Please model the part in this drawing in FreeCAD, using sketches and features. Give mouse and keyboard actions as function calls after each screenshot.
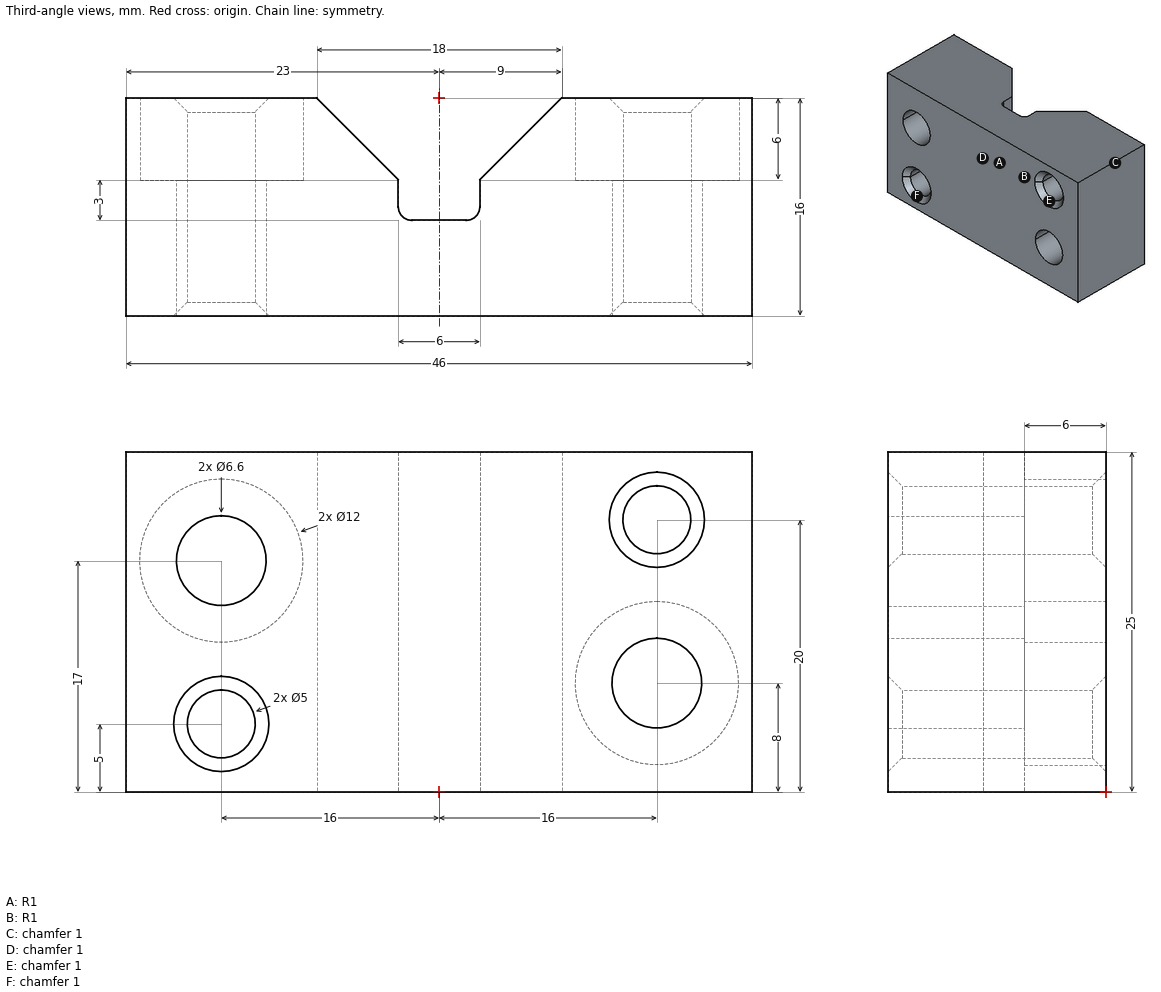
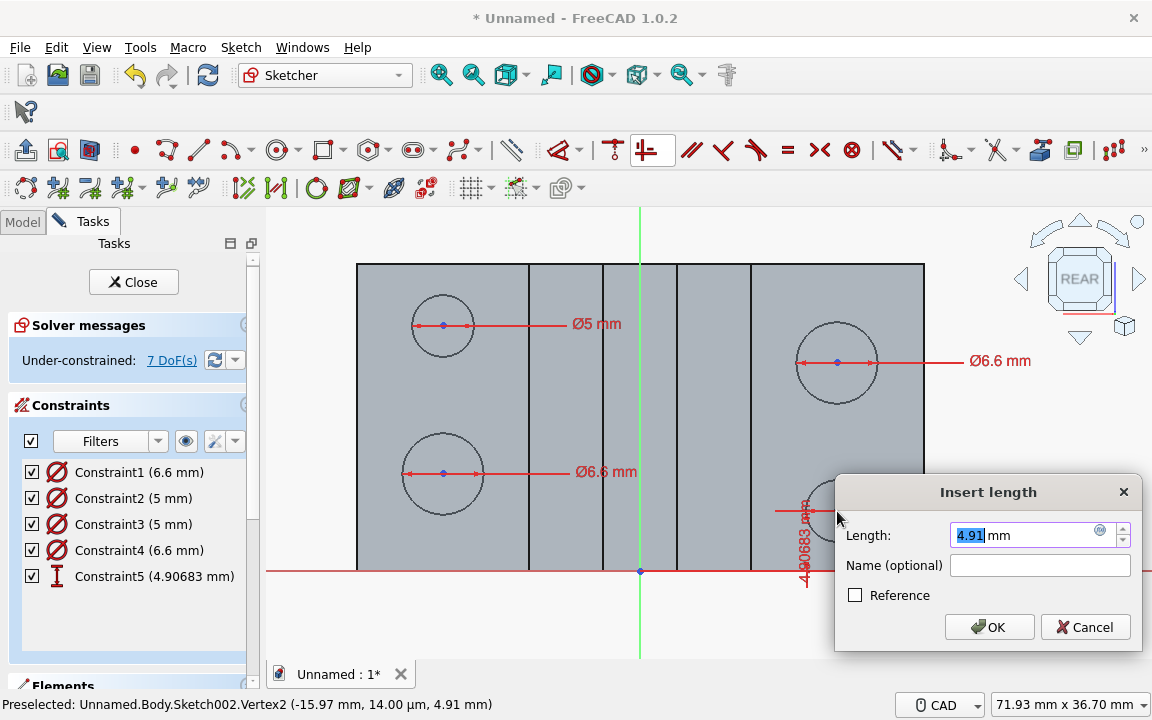
text(5)
key(Return)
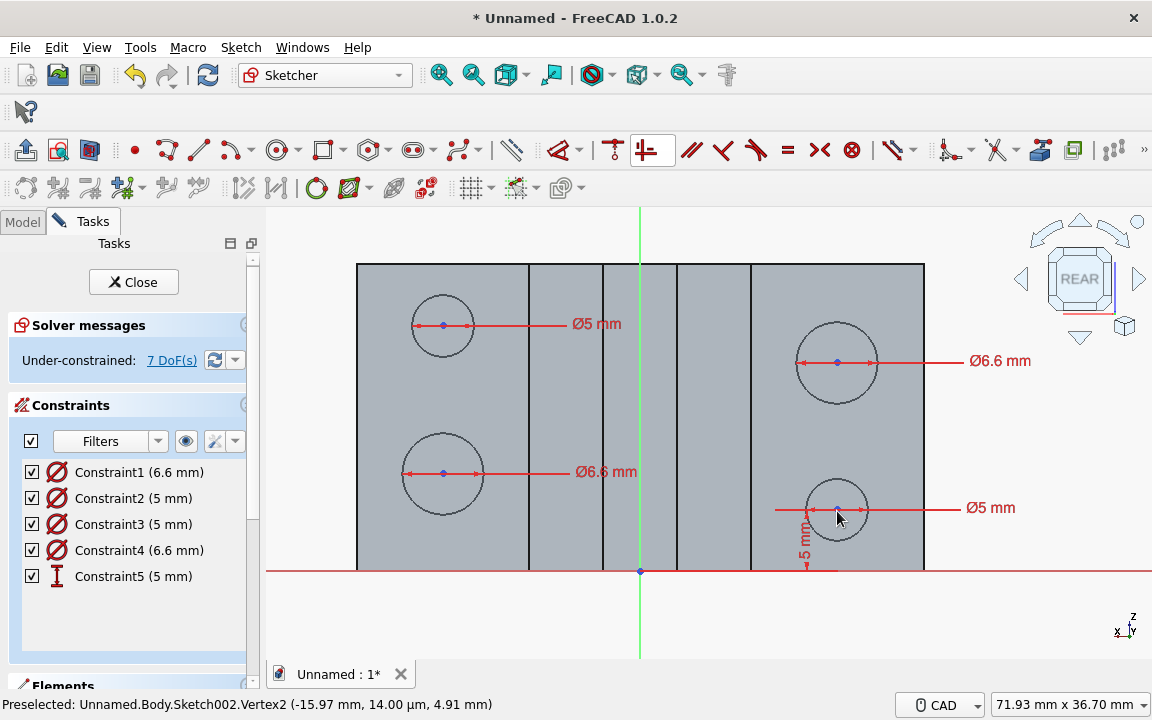
click(443, 474)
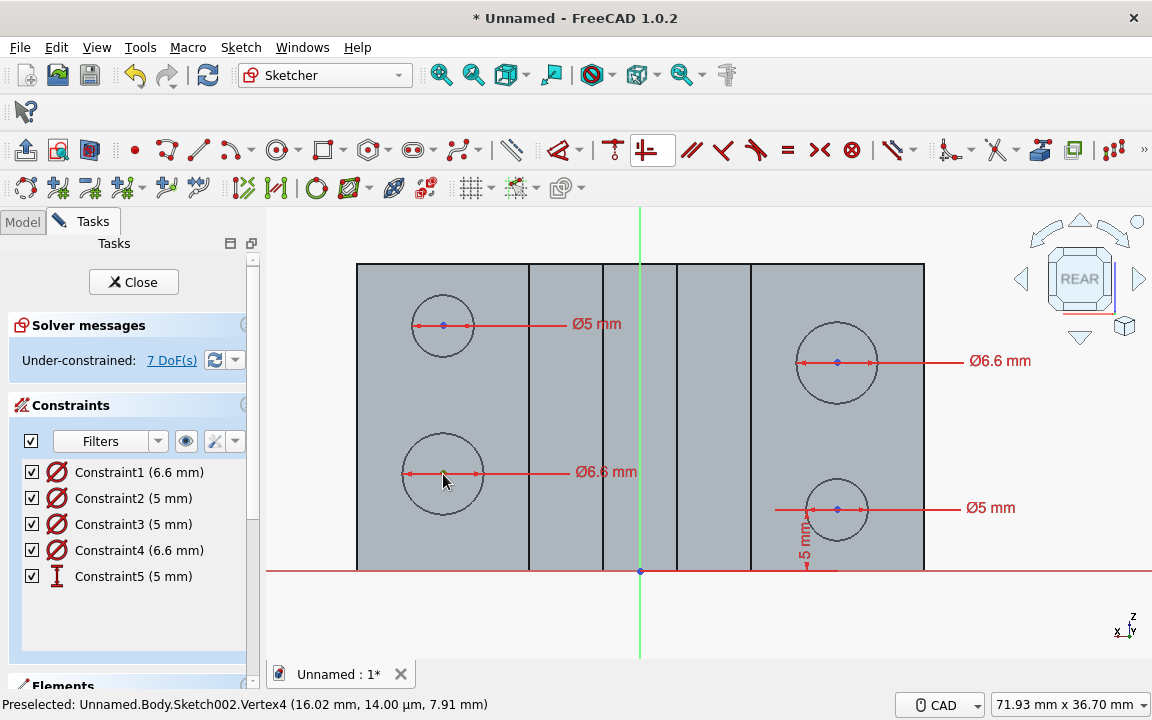
key(i)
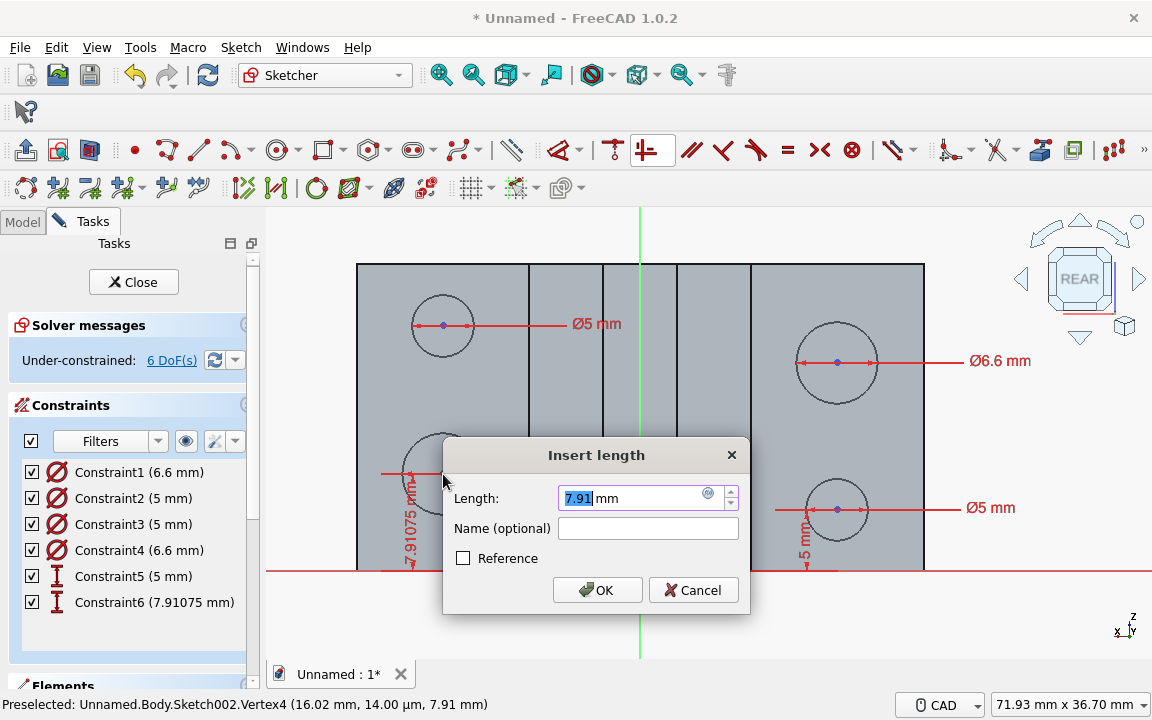
text(8)
key(Return)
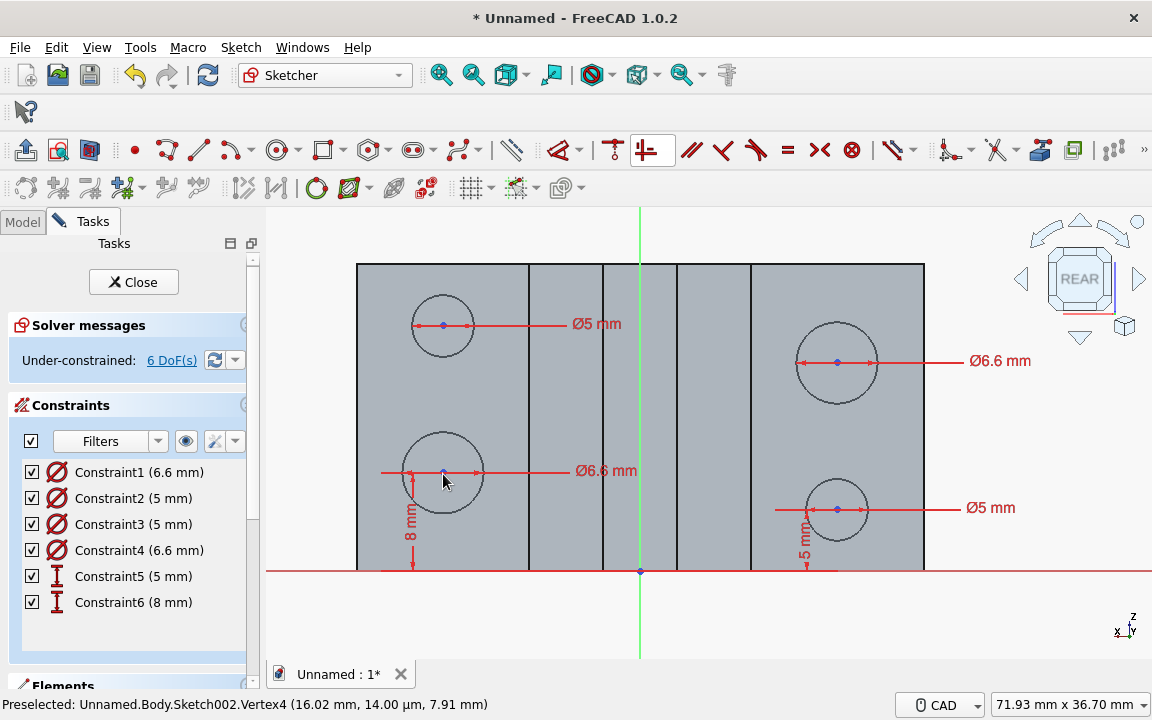
click(837, 363)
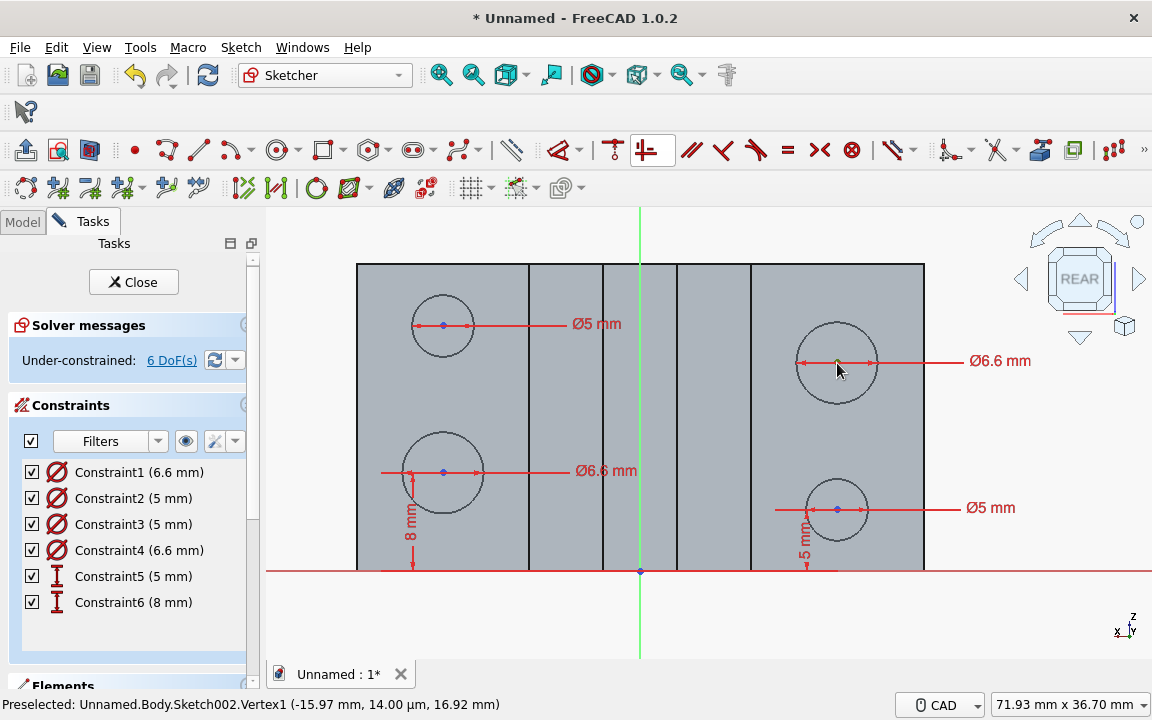
click(582, 150)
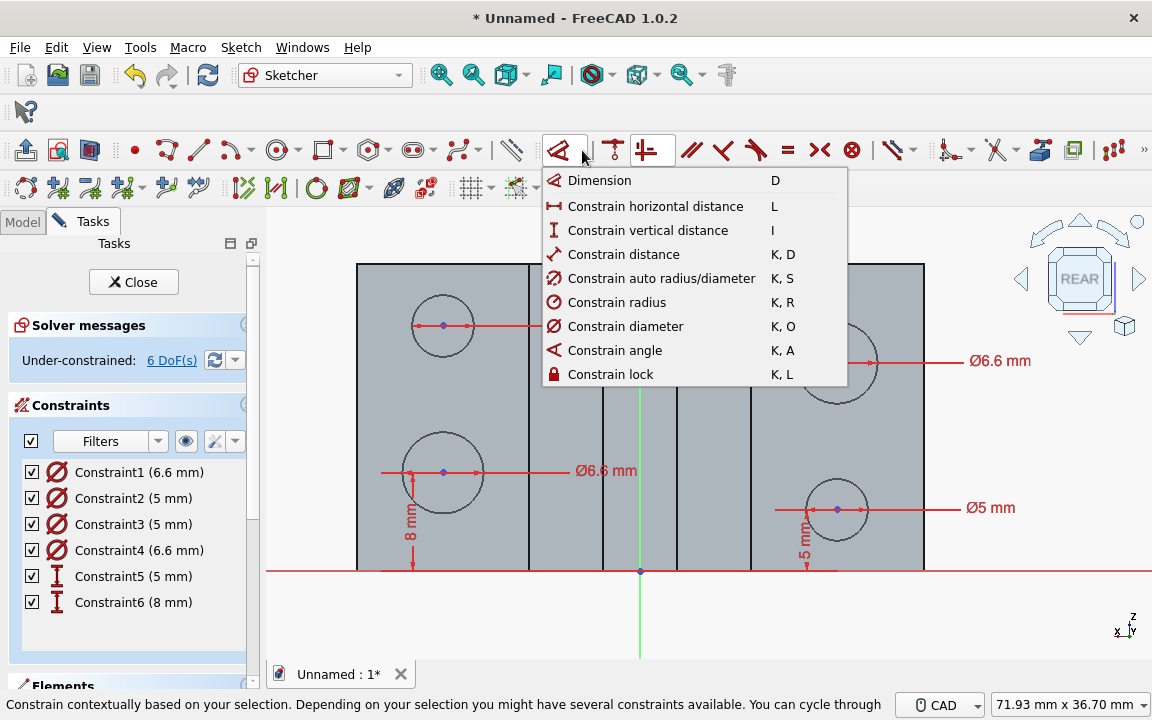
click(695, 206)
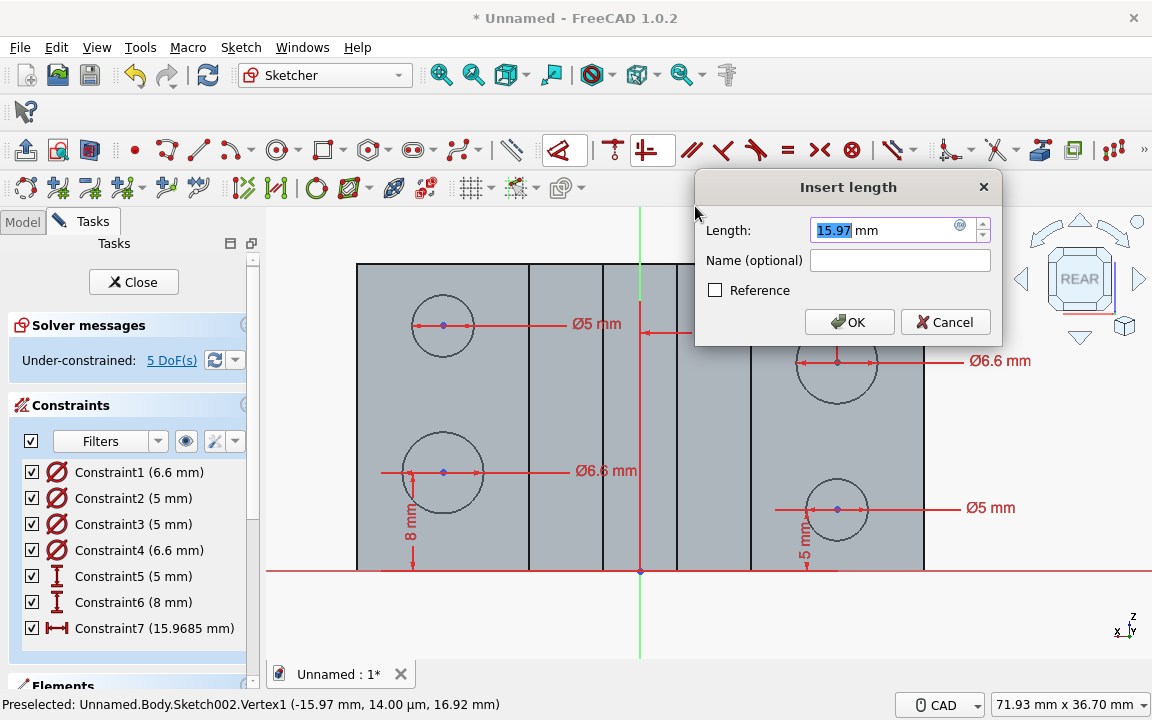
text(16)
key(Return)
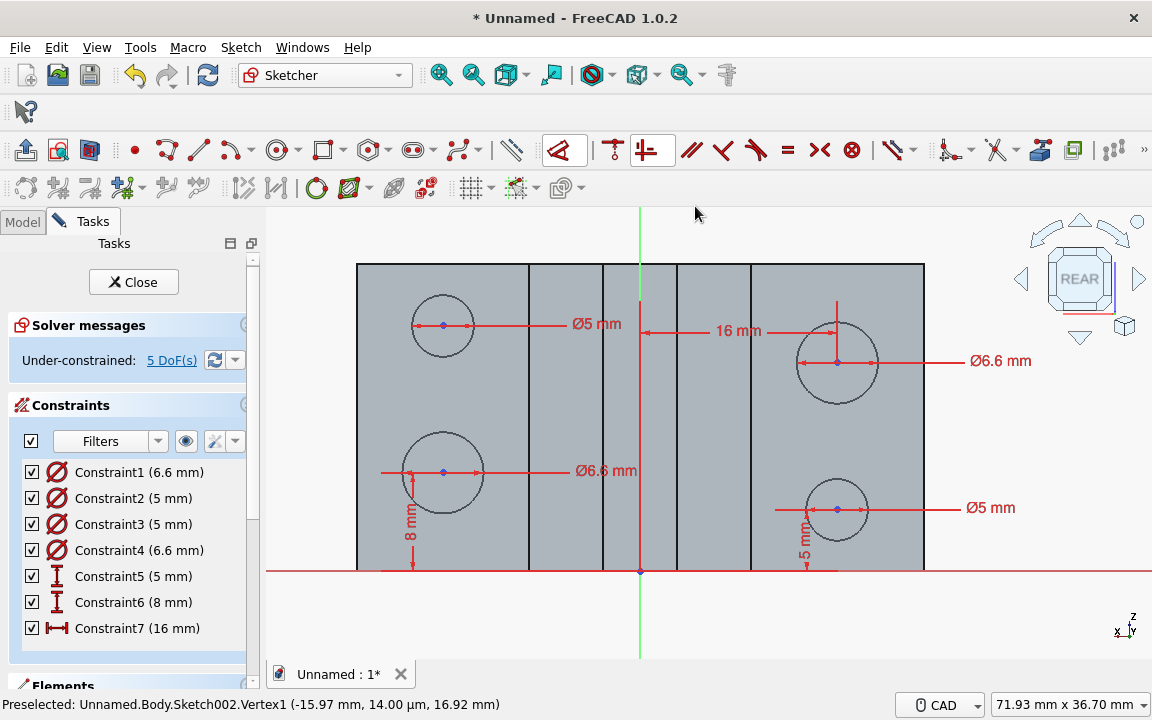
click(837, 363)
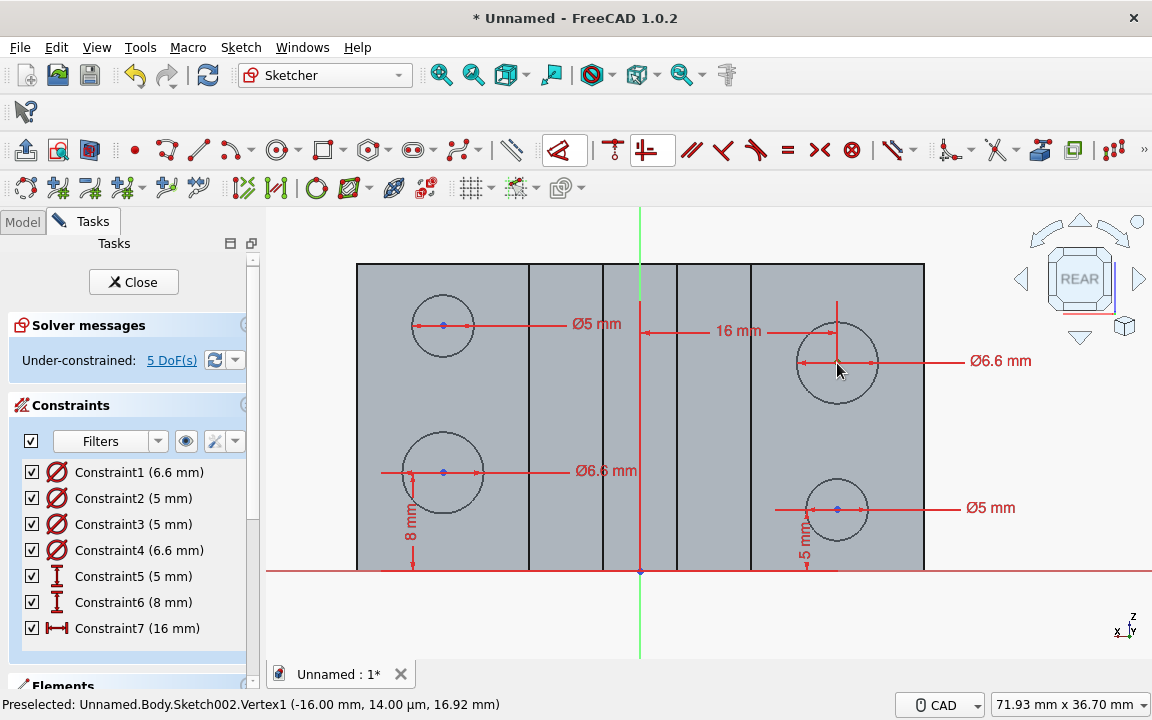
key(i)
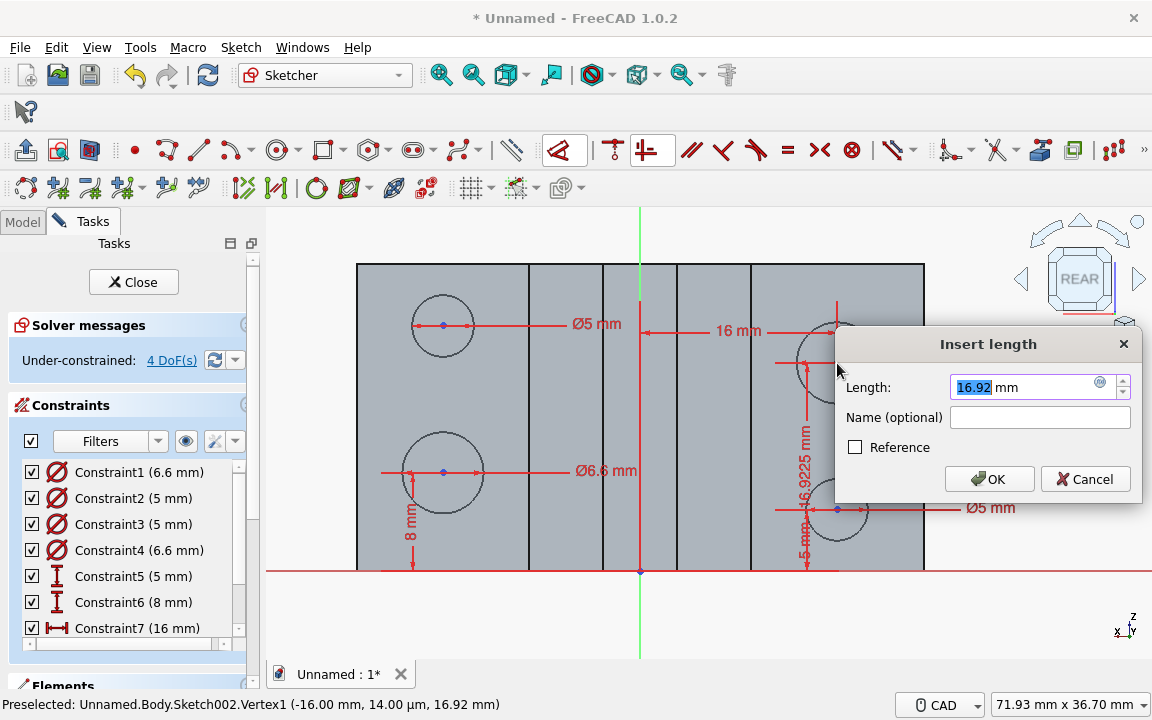
text(17)
key(Return)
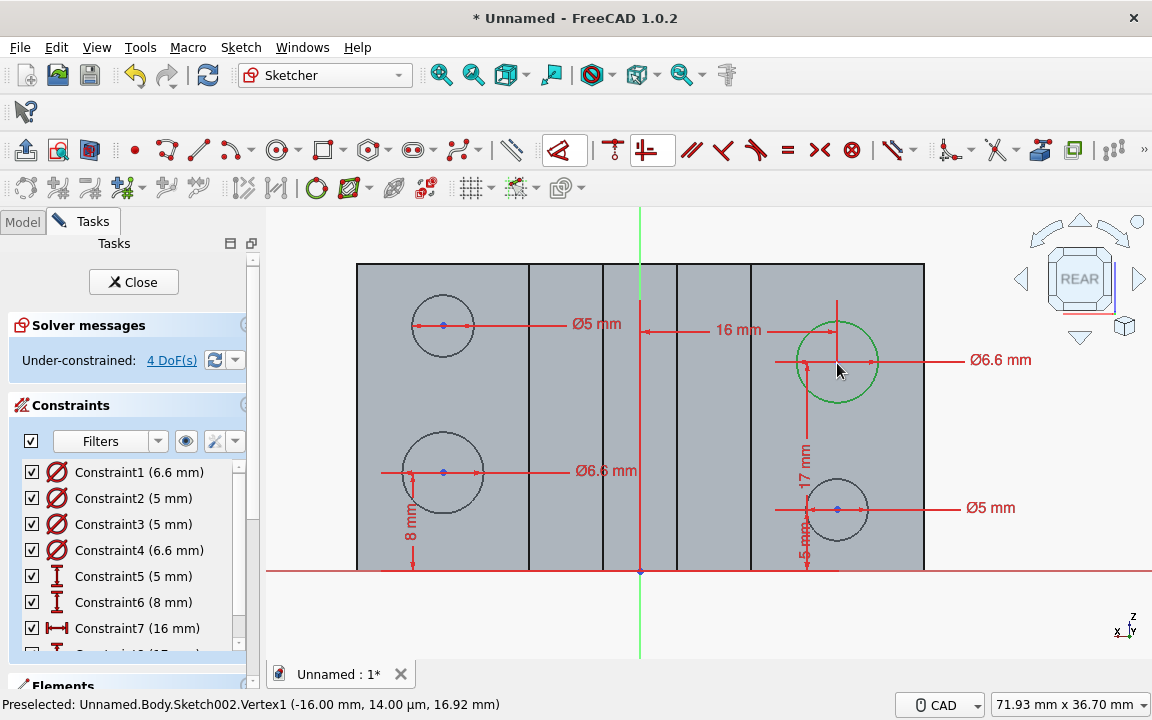
click(837, 510)